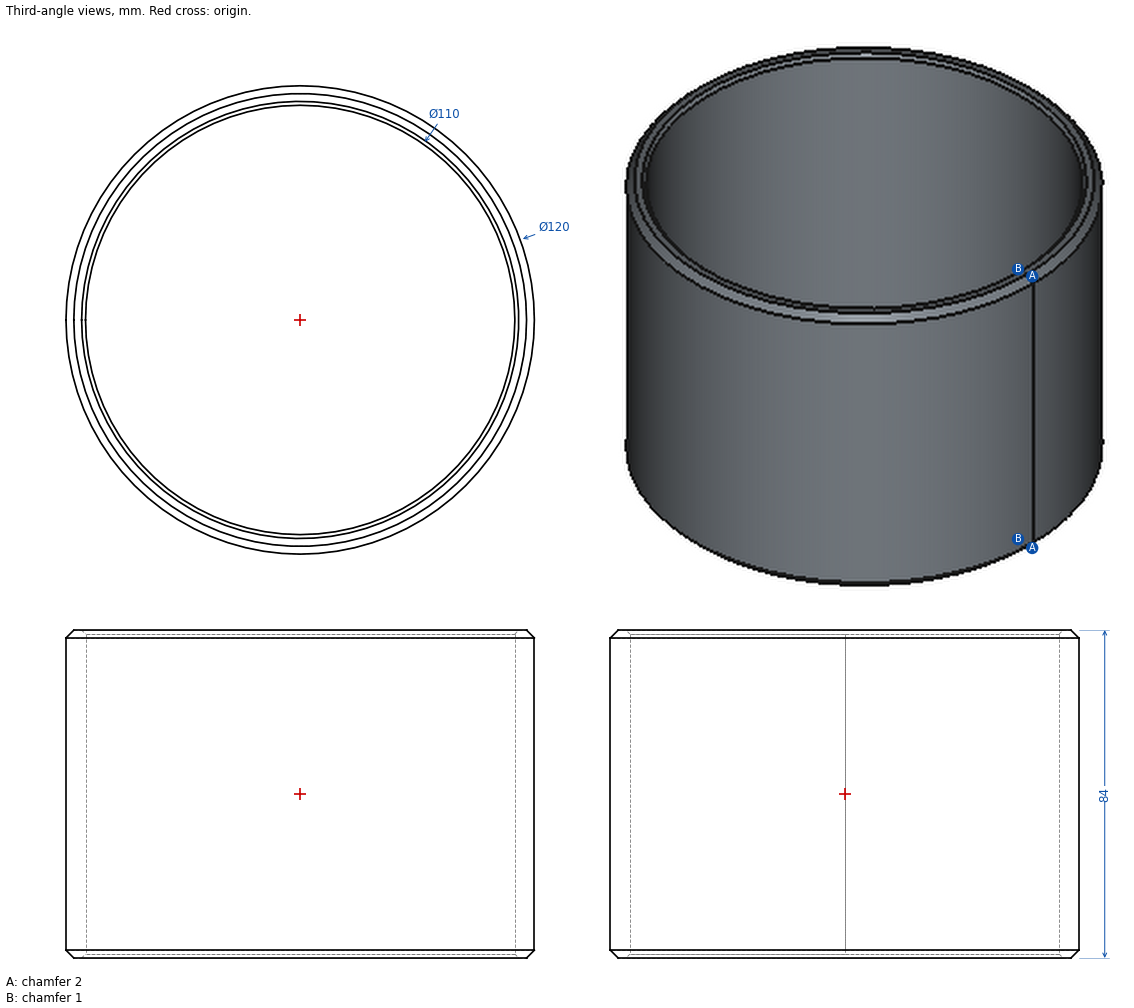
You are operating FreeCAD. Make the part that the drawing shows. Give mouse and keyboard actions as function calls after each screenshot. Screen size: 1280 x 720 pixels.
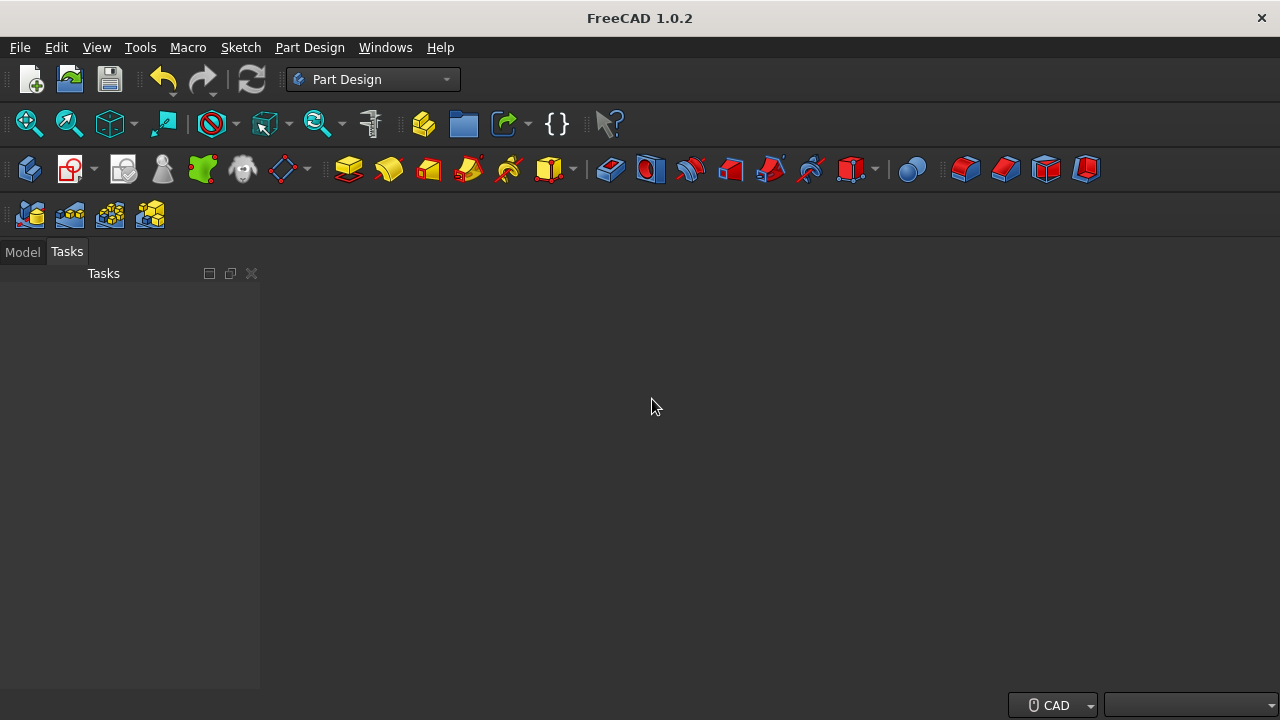
click(30, 80)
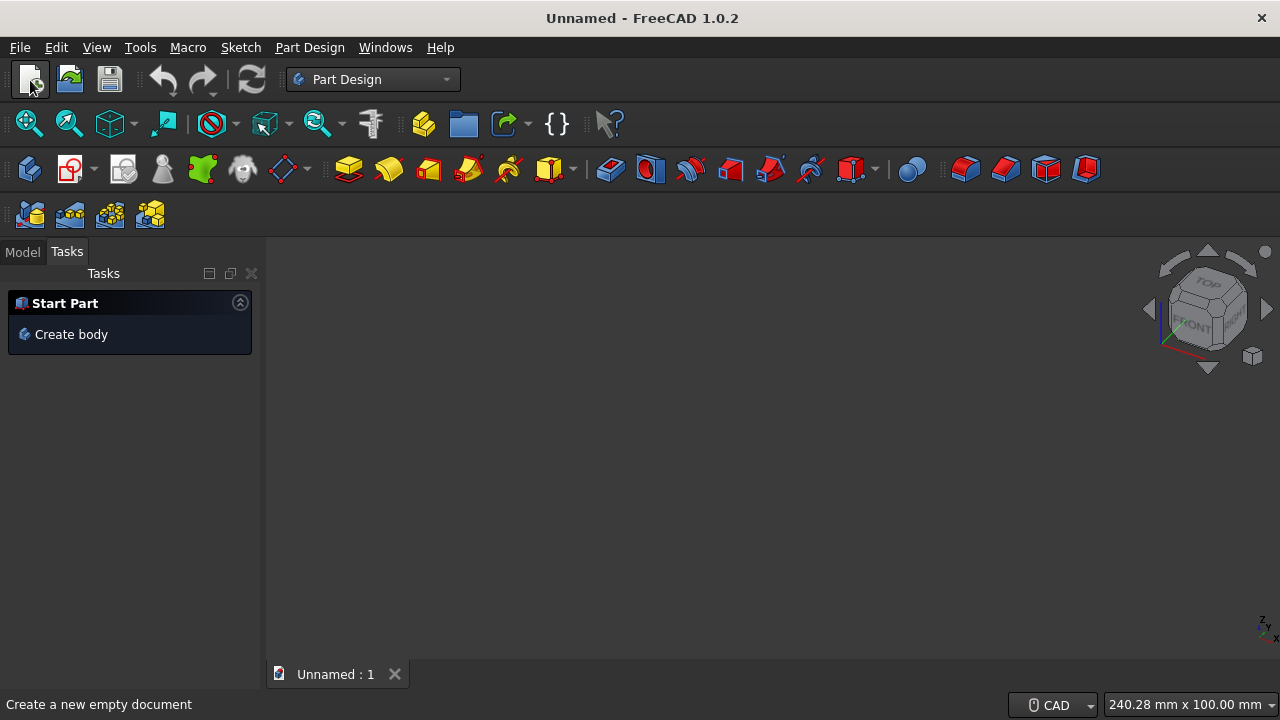
click(70, 170)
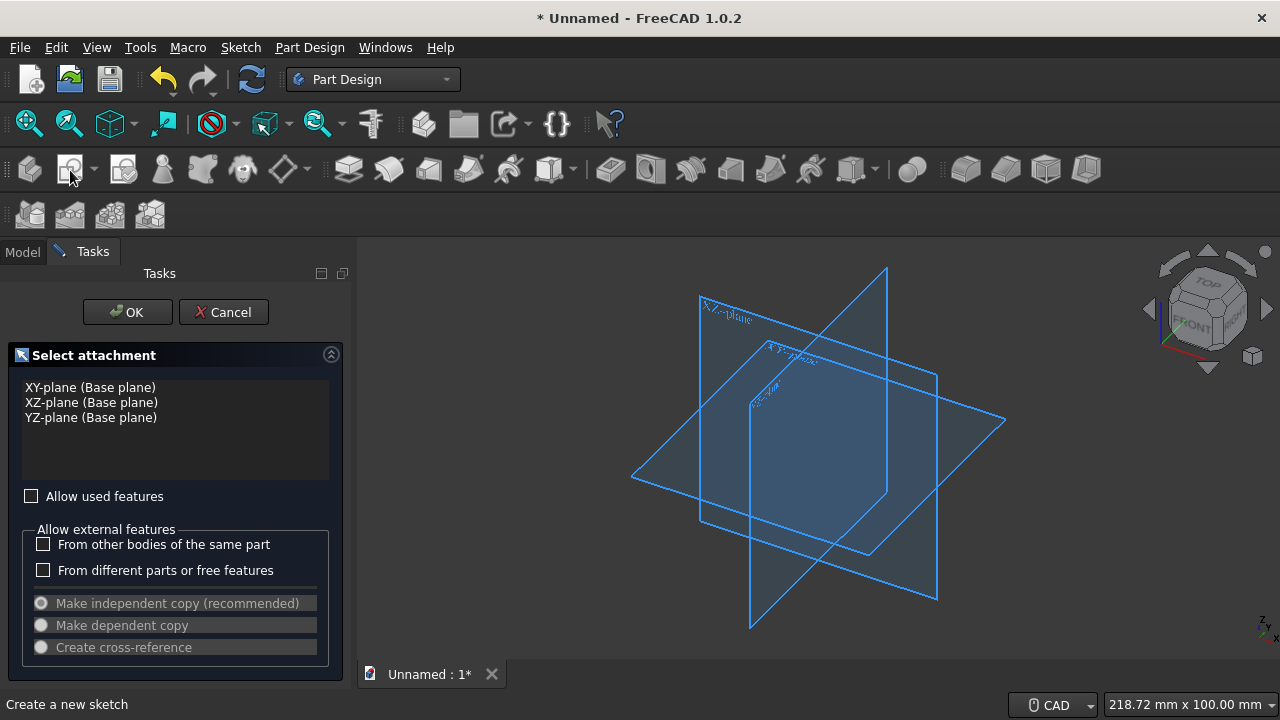
click(82, 388)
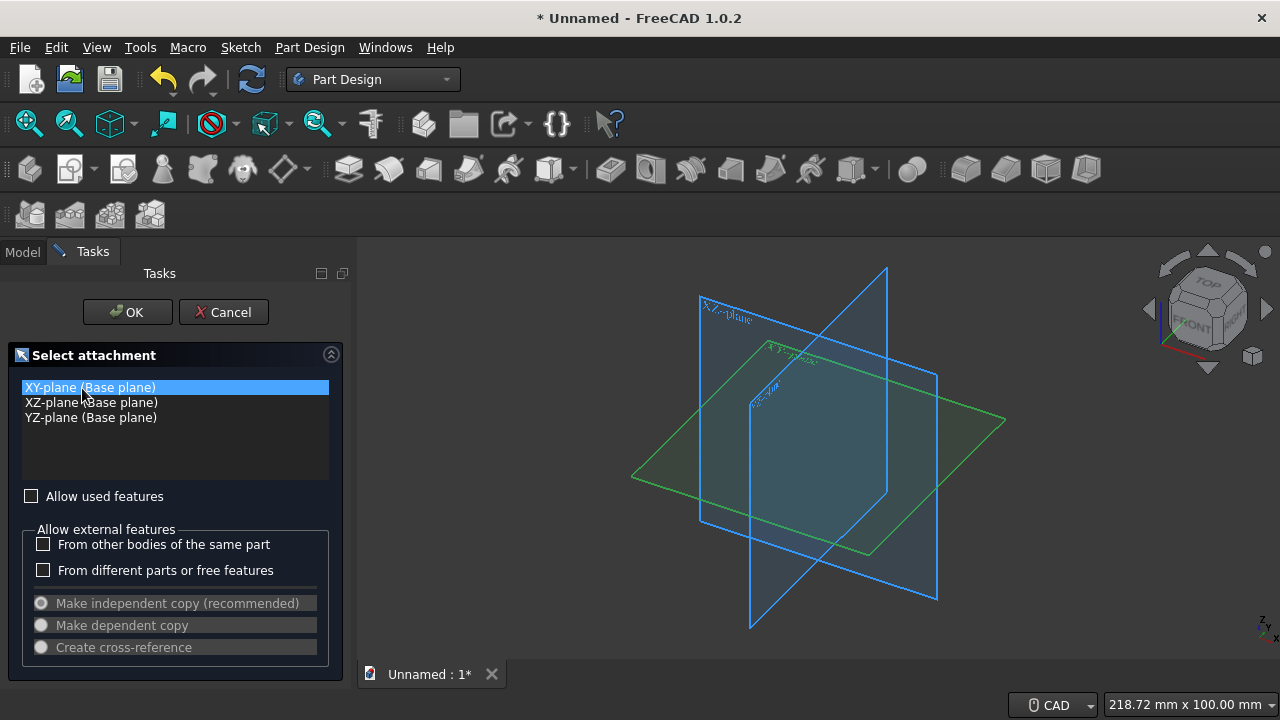
click(128, 312)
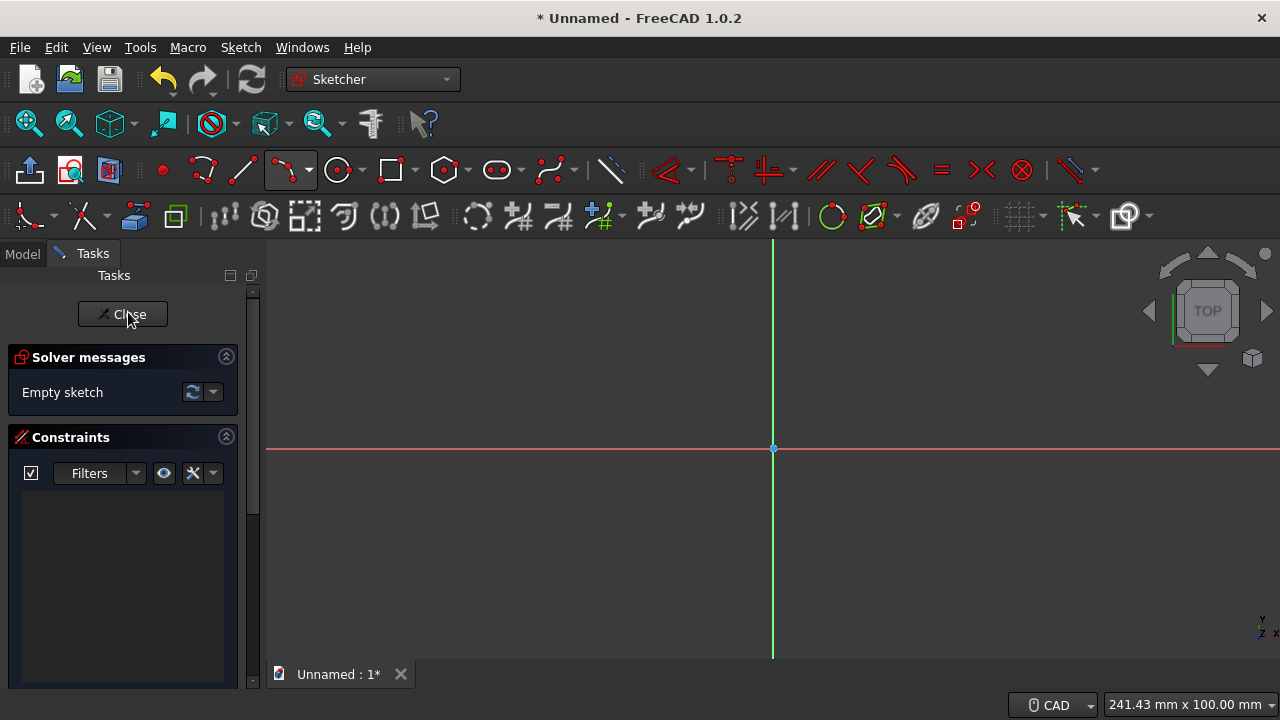
scroll(621, 449, down, 3)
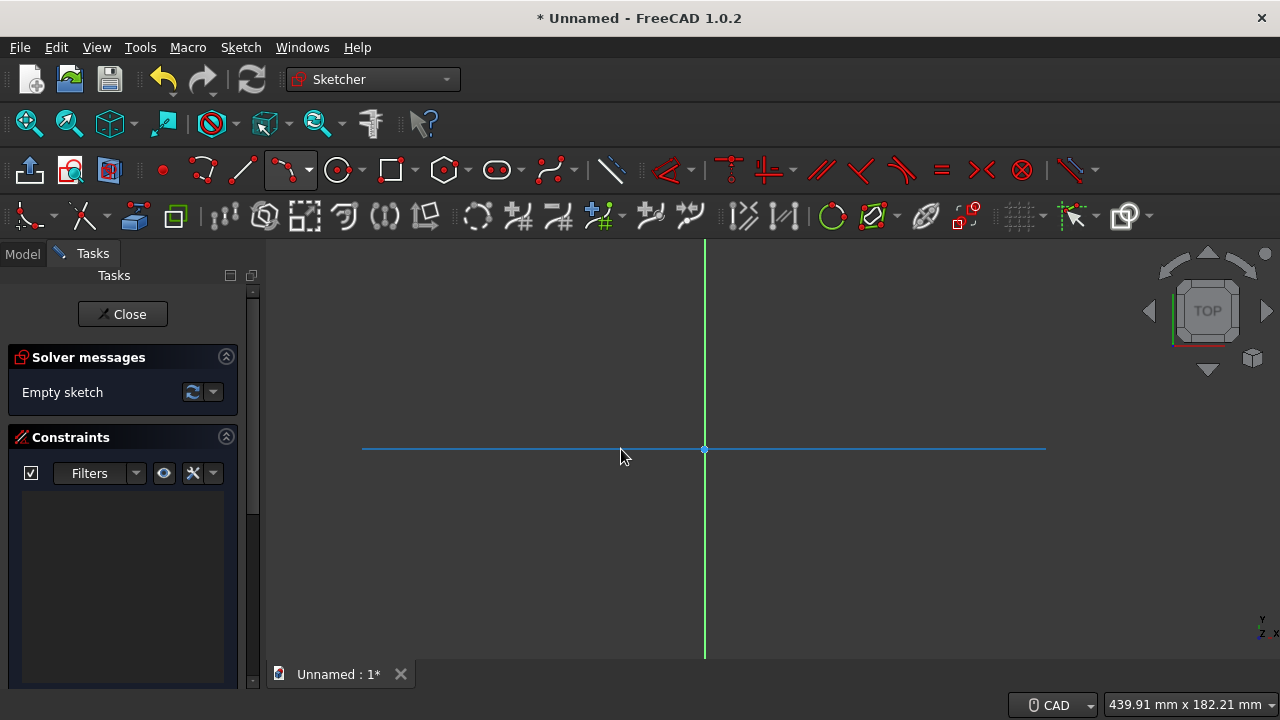
click(338, 170)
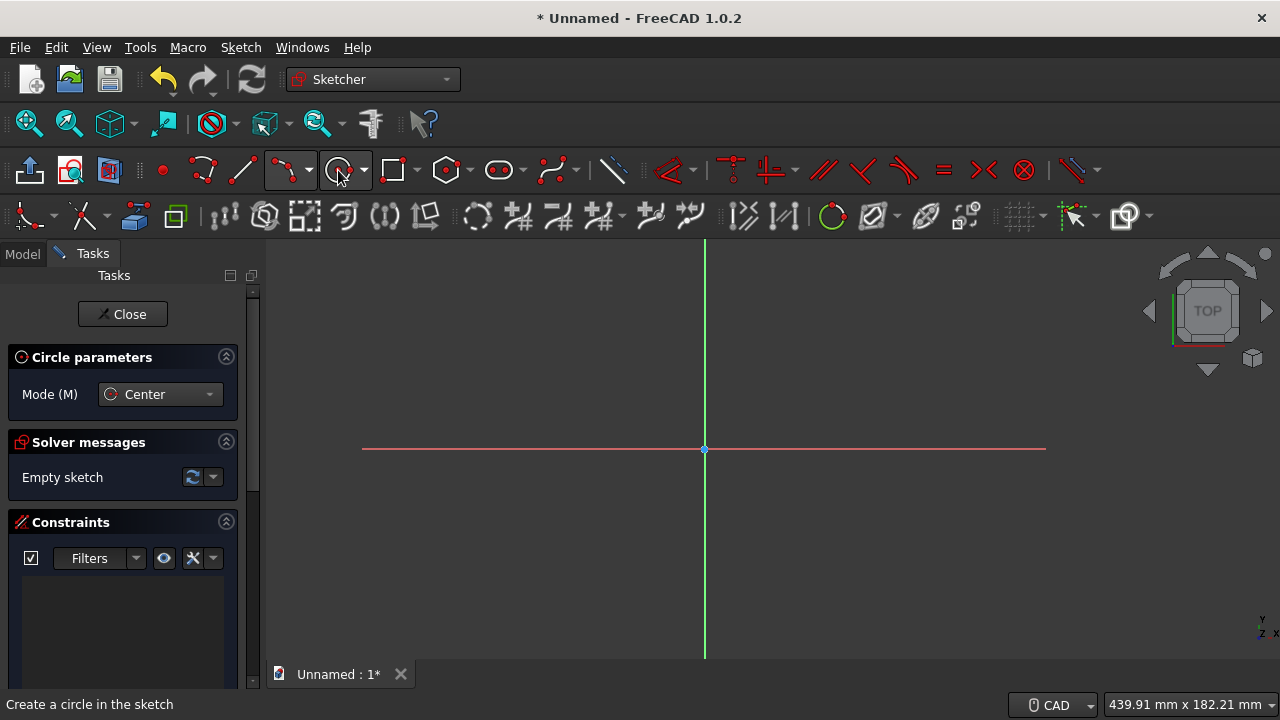
click(705, 449)
click(802, 351)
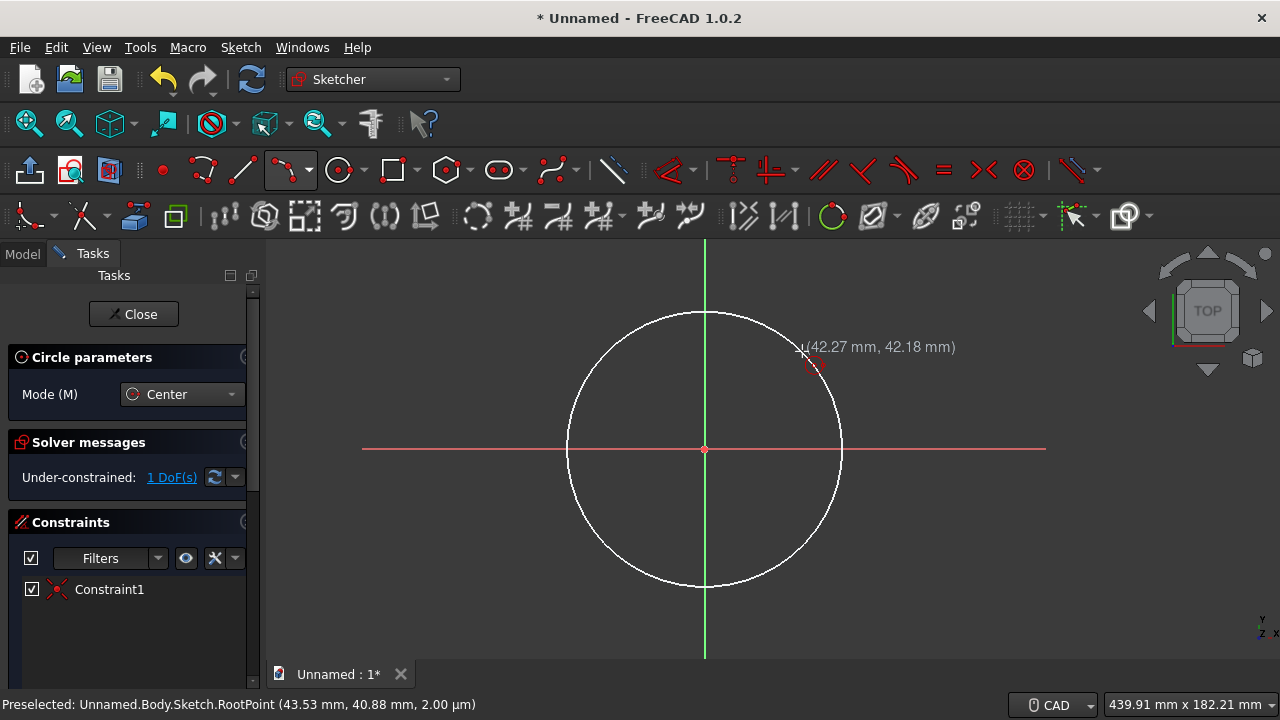
click(705, 449)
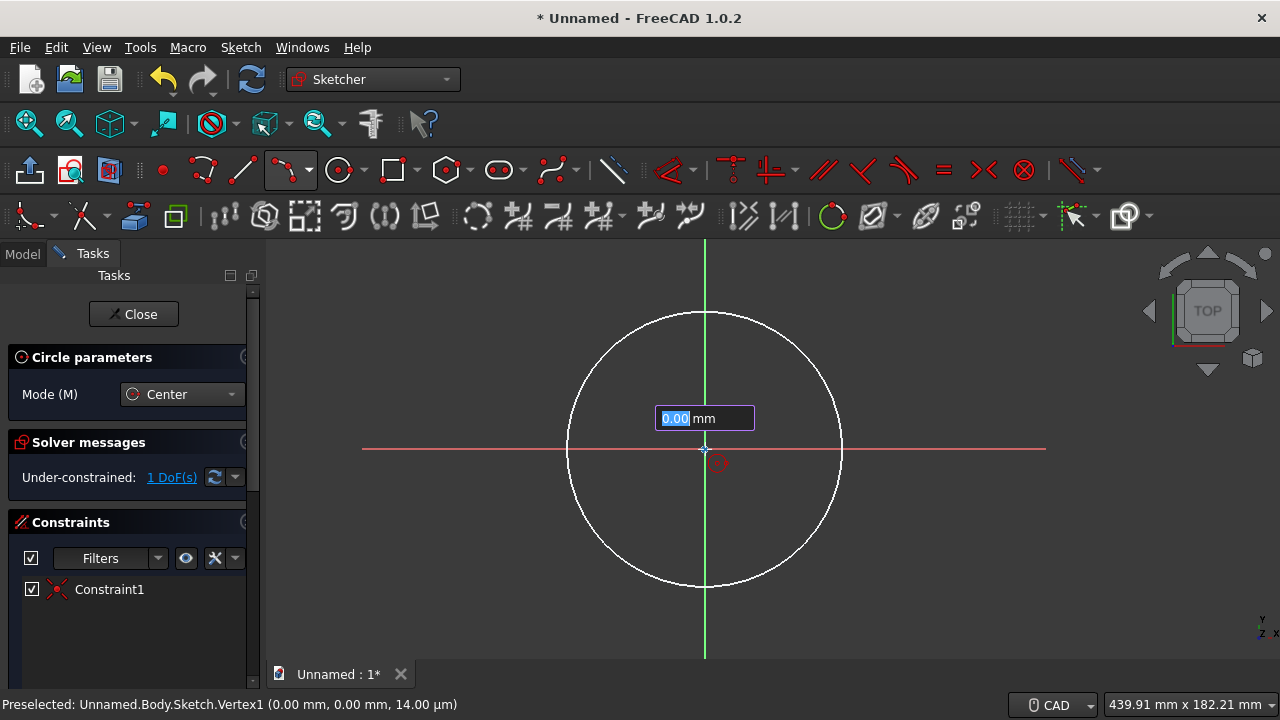
scroll(794, 360, up, 2)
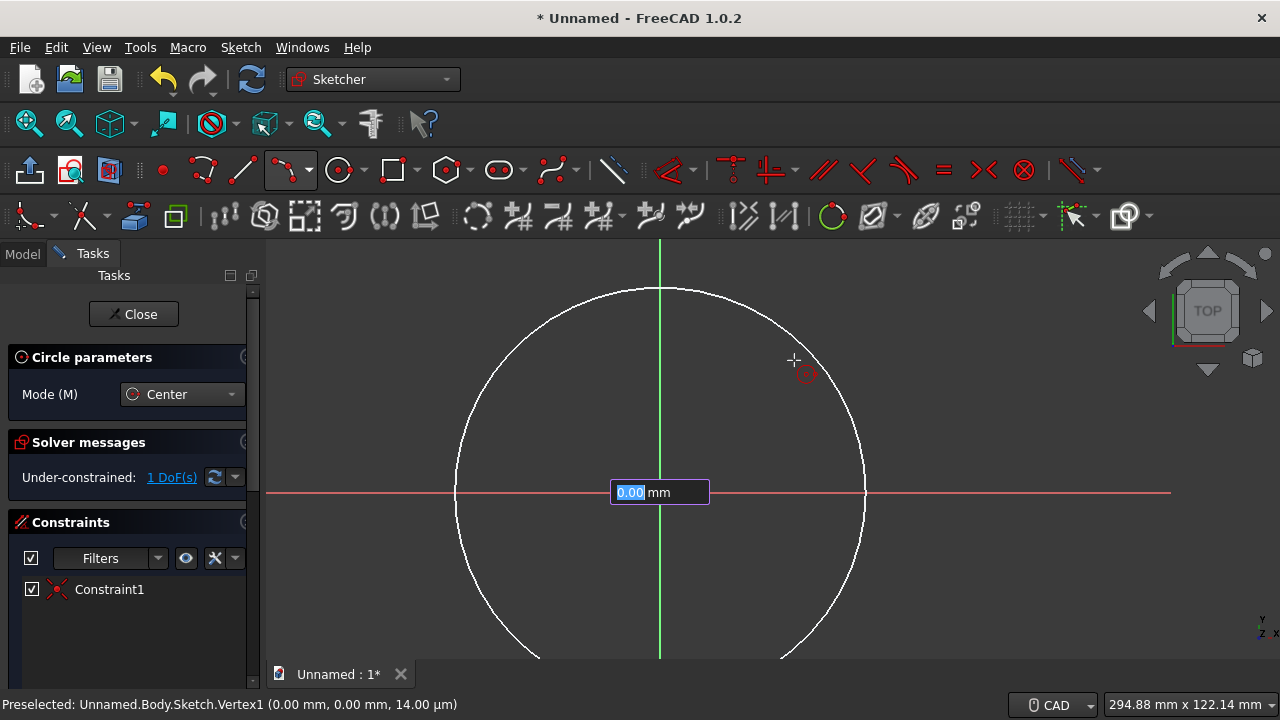
click(794, 359)
key(Escape)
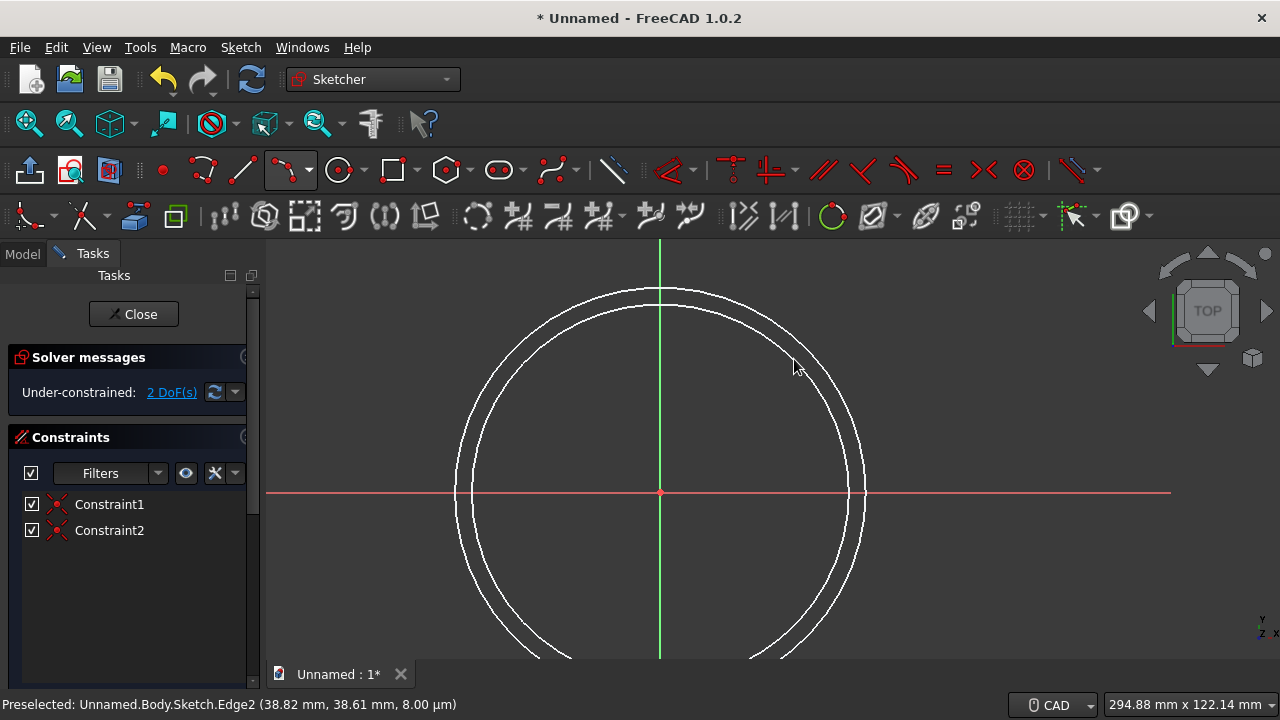
click(668, 170)